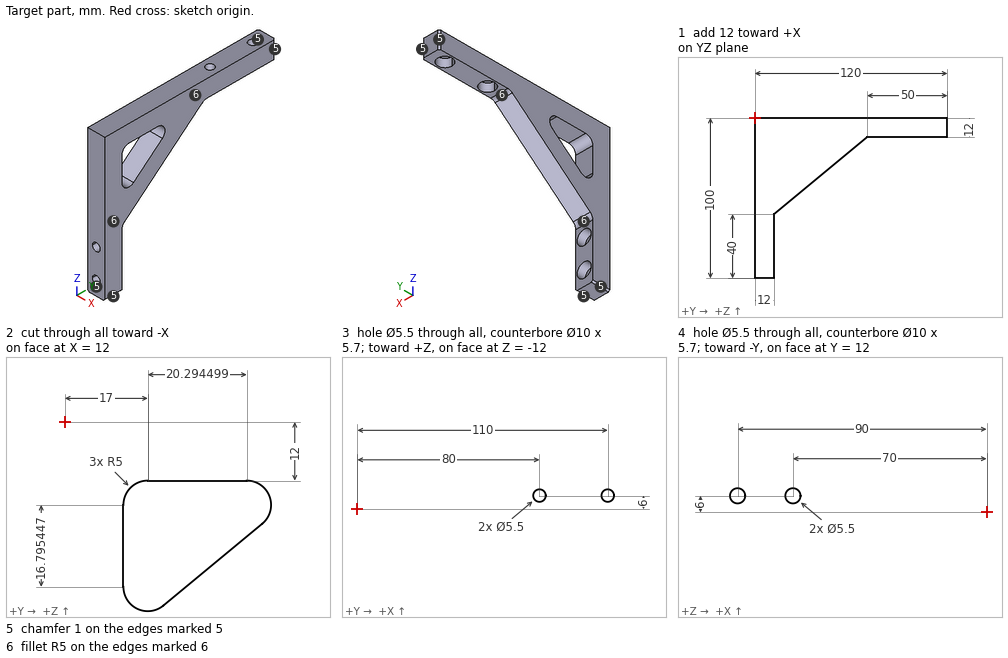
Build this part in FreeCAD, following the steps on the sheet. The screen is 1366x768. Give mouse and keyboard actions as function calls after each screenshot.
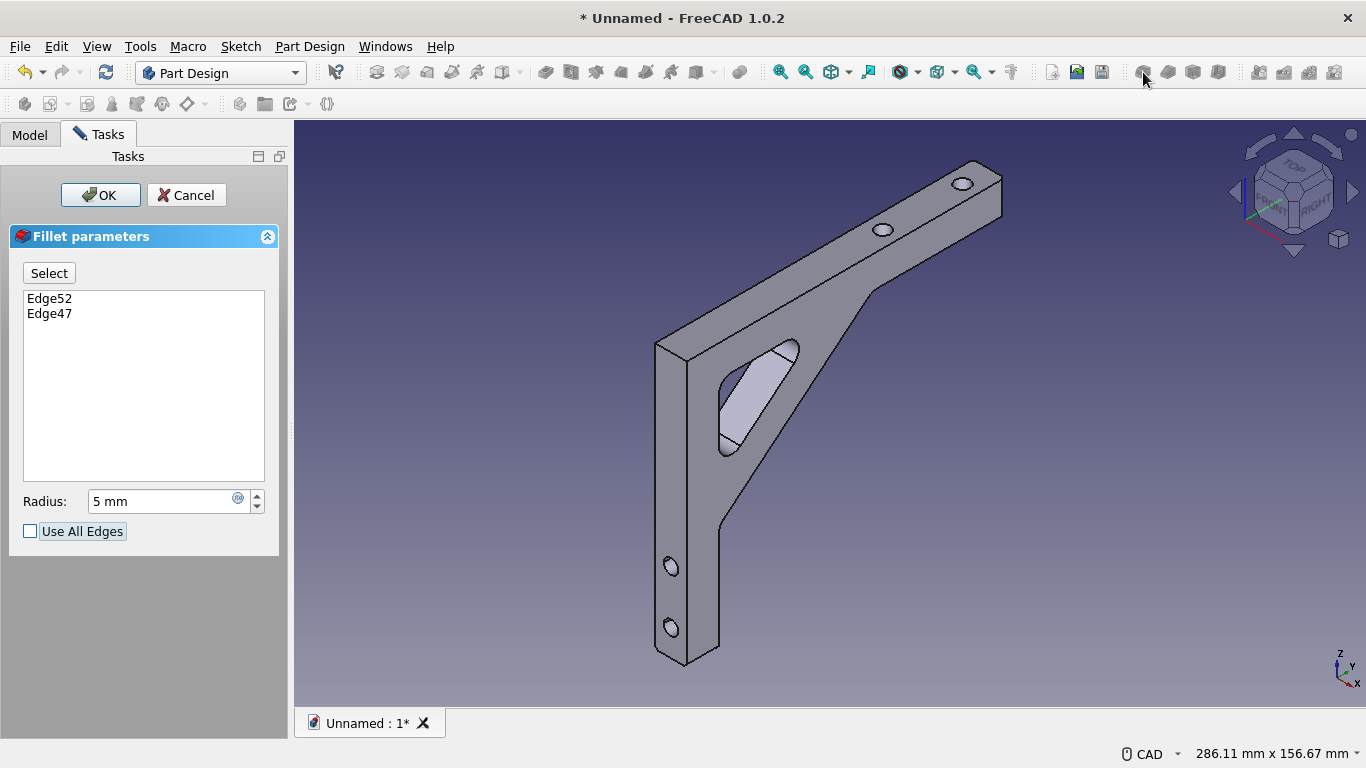
click(101, 195)